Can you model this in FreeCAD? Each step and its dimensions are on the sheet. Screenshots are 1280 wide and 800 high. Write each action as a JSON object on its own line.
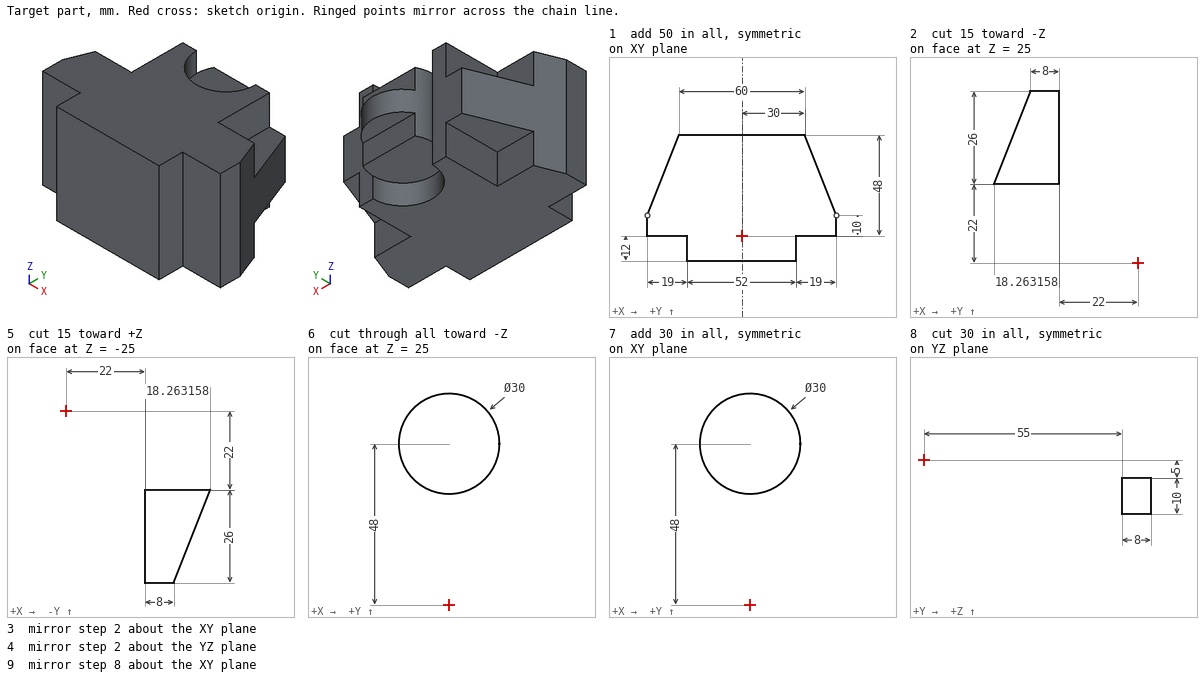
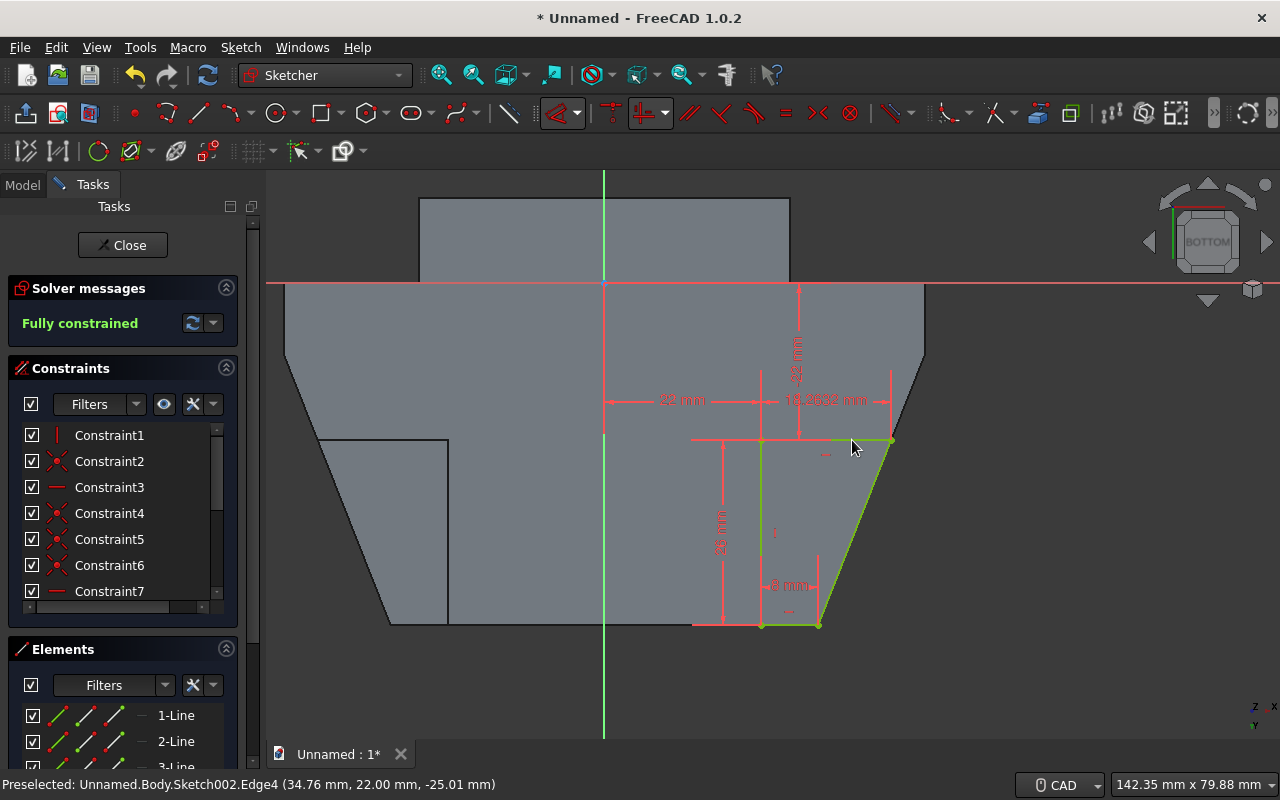
{"action": "left_click", "coordinate": [123, 245]}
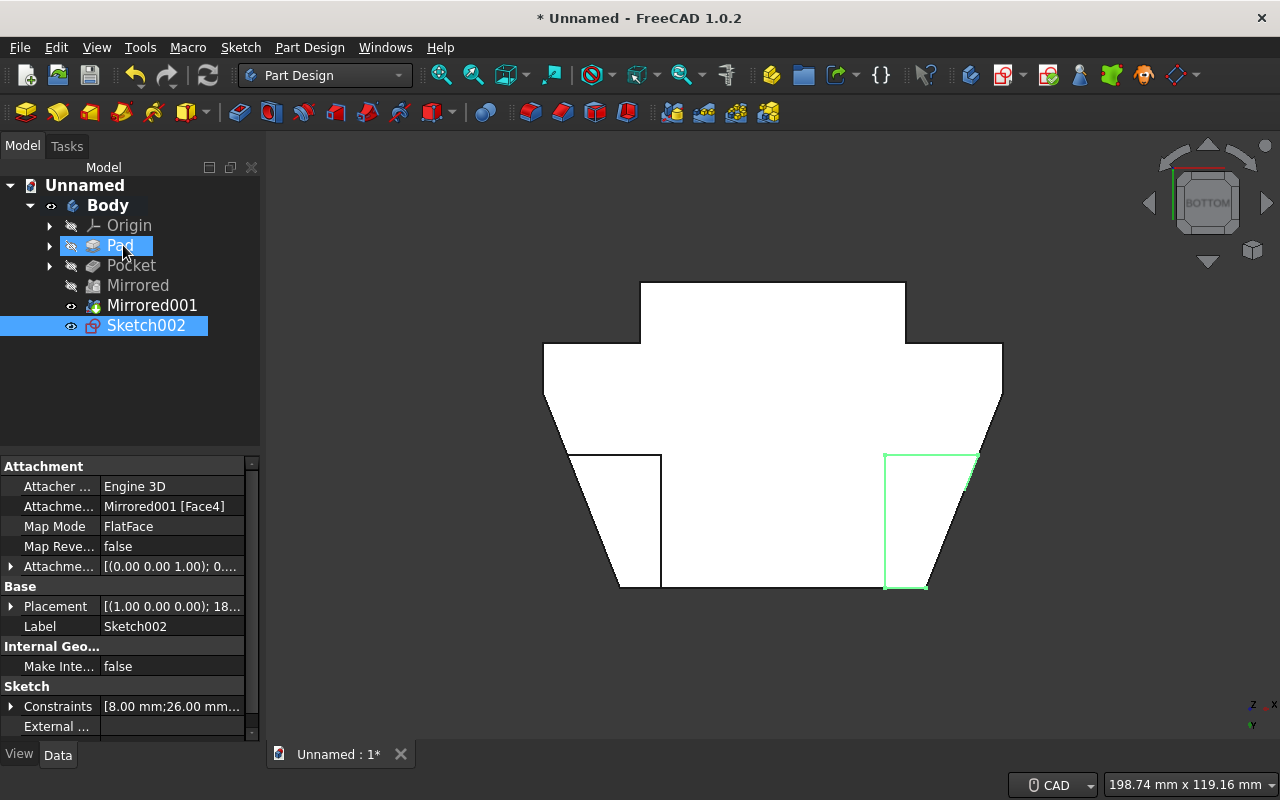
{"action": "left_click", "coordinate": [240, 112]}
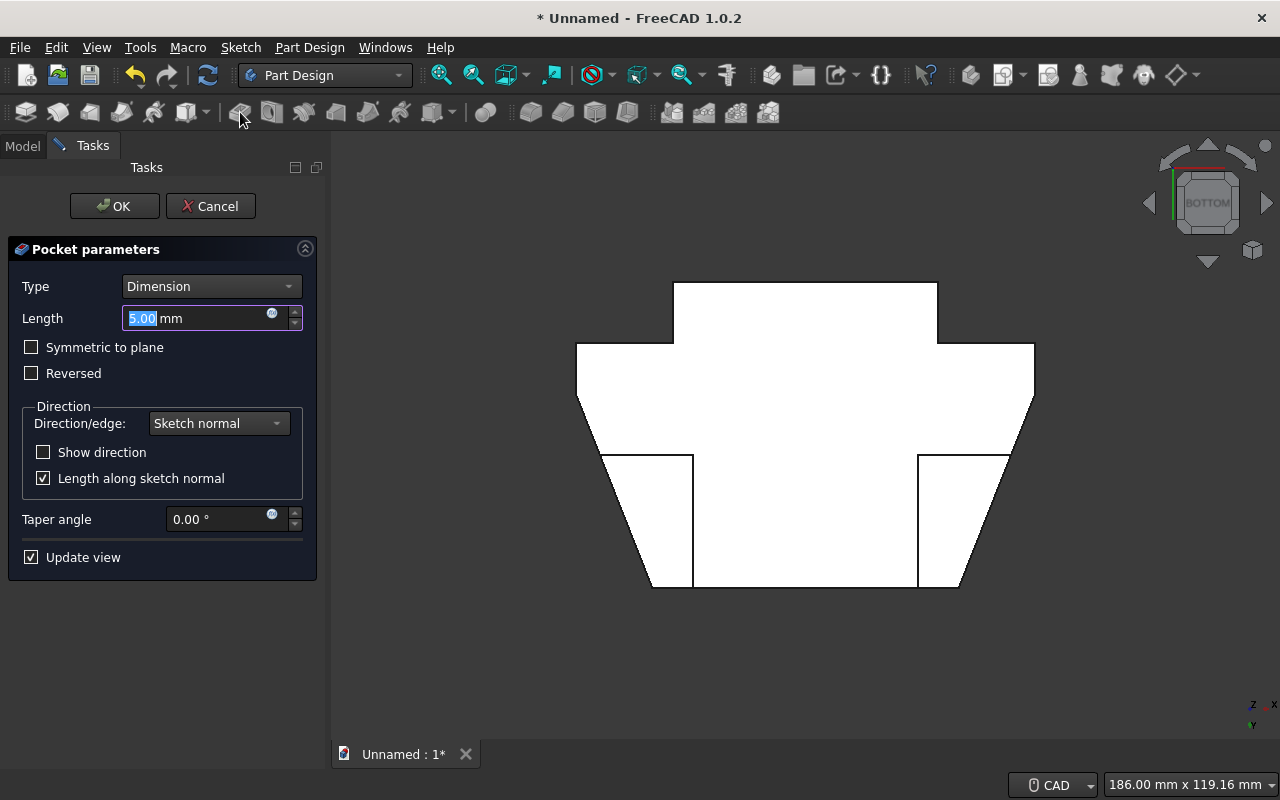
{"action": "type", "text": "15"}
{"action": "key", "text": "Tab"}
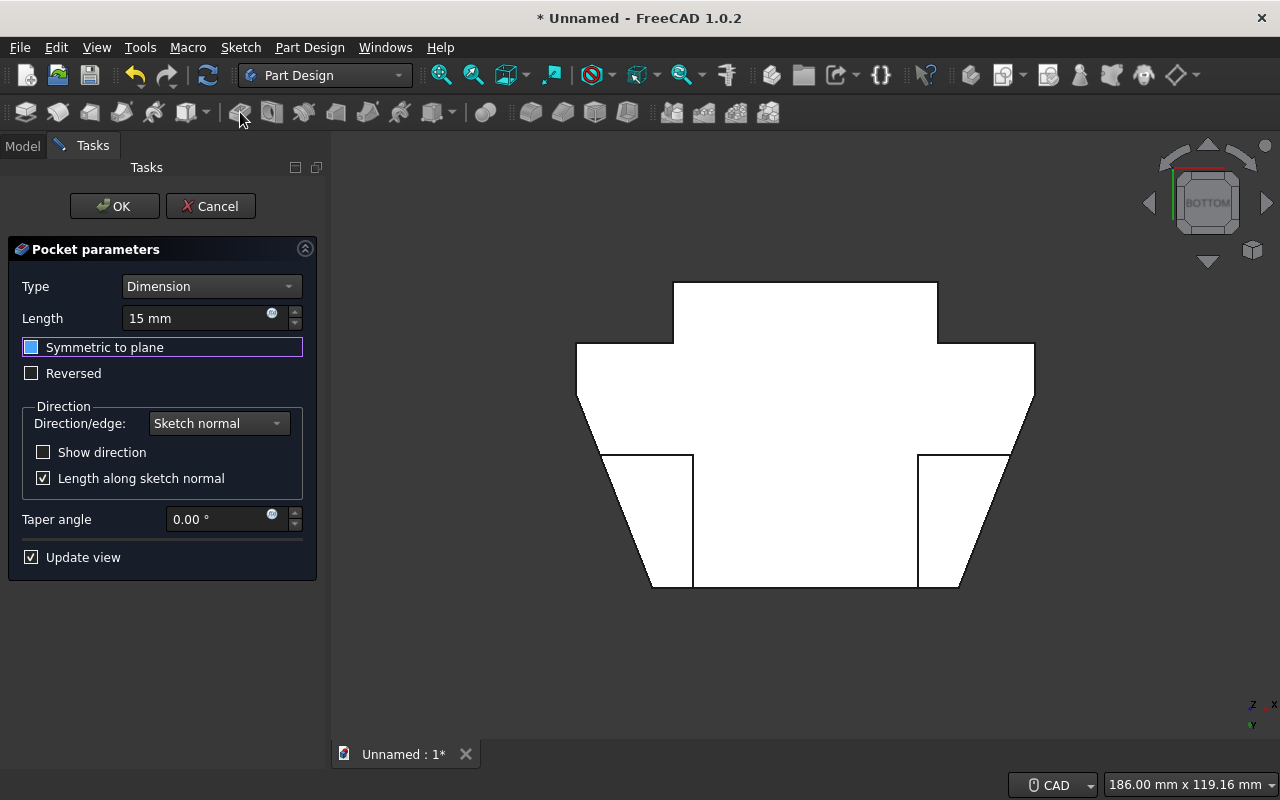
{"action": "left_click", "coordinate": [115, 206]}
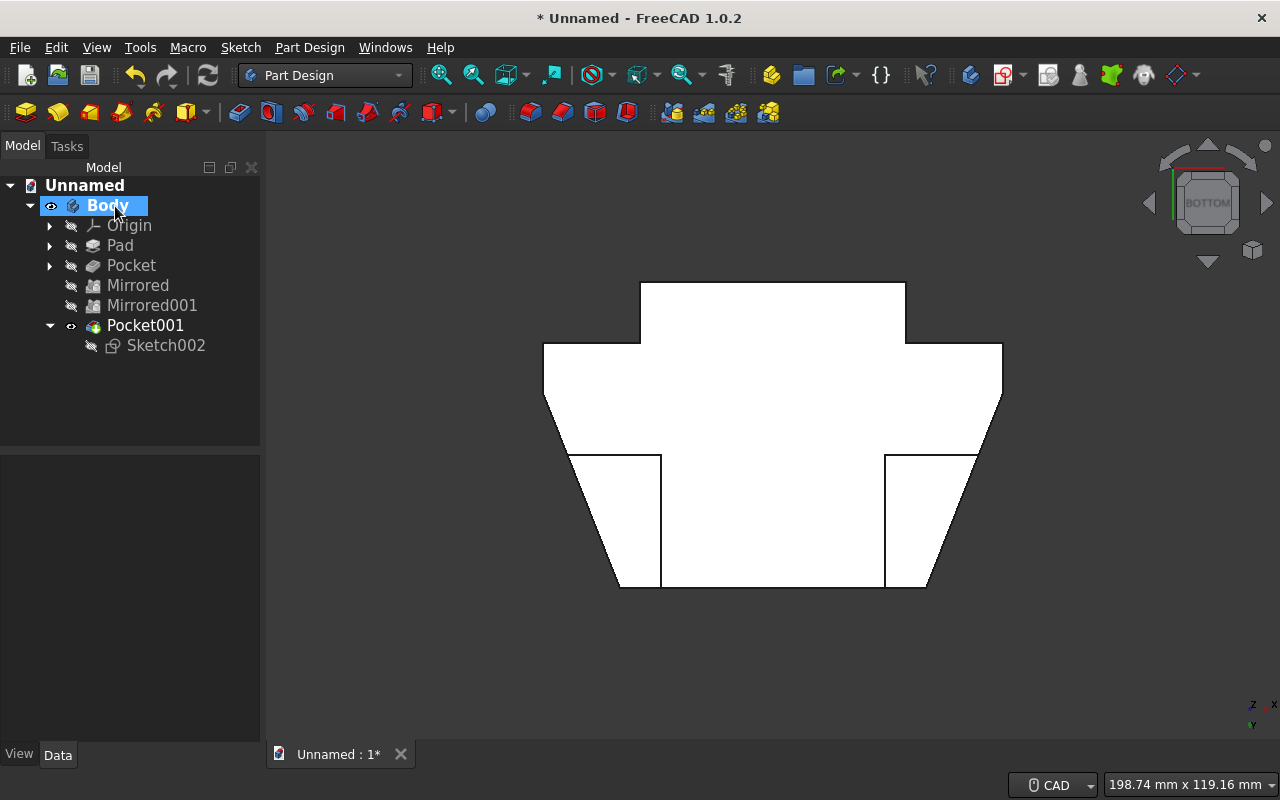
{"action": "key", "text": "0"}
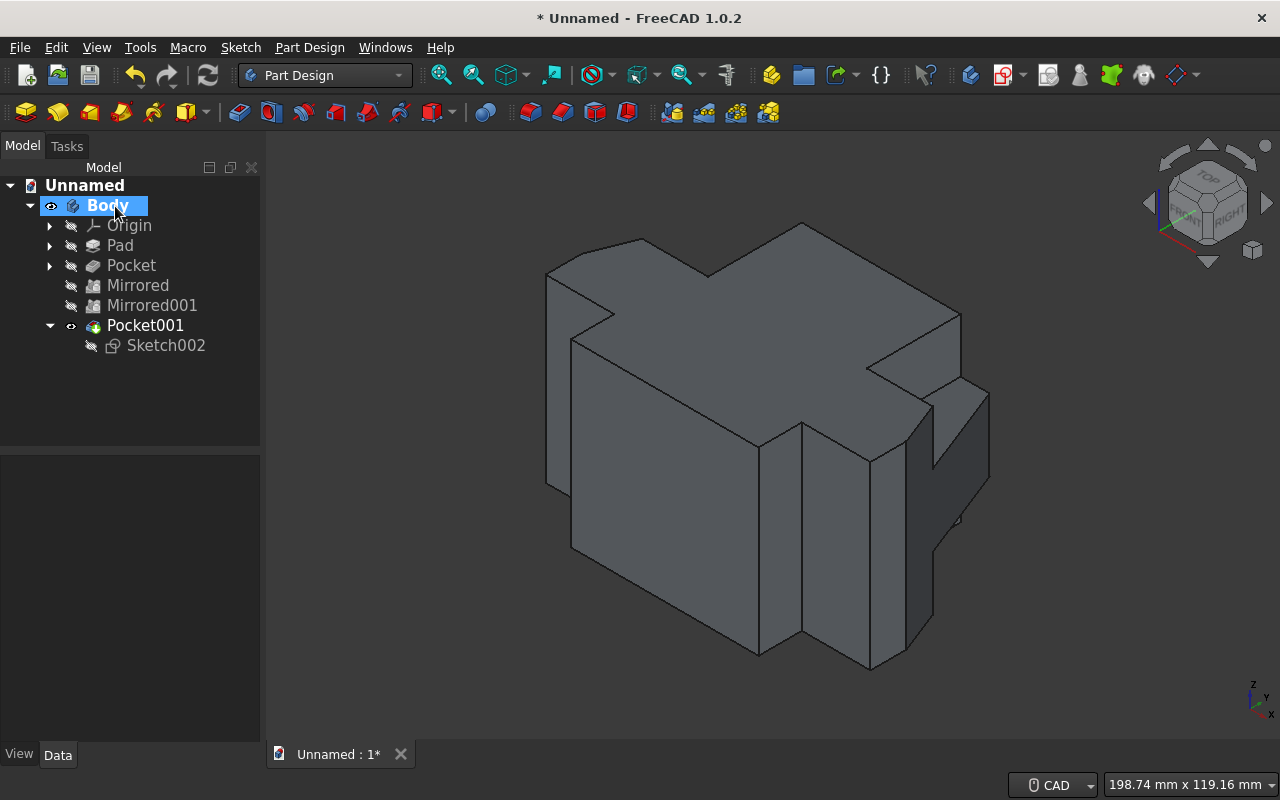
{"action": "left_click", "coordinate": [773, 330]}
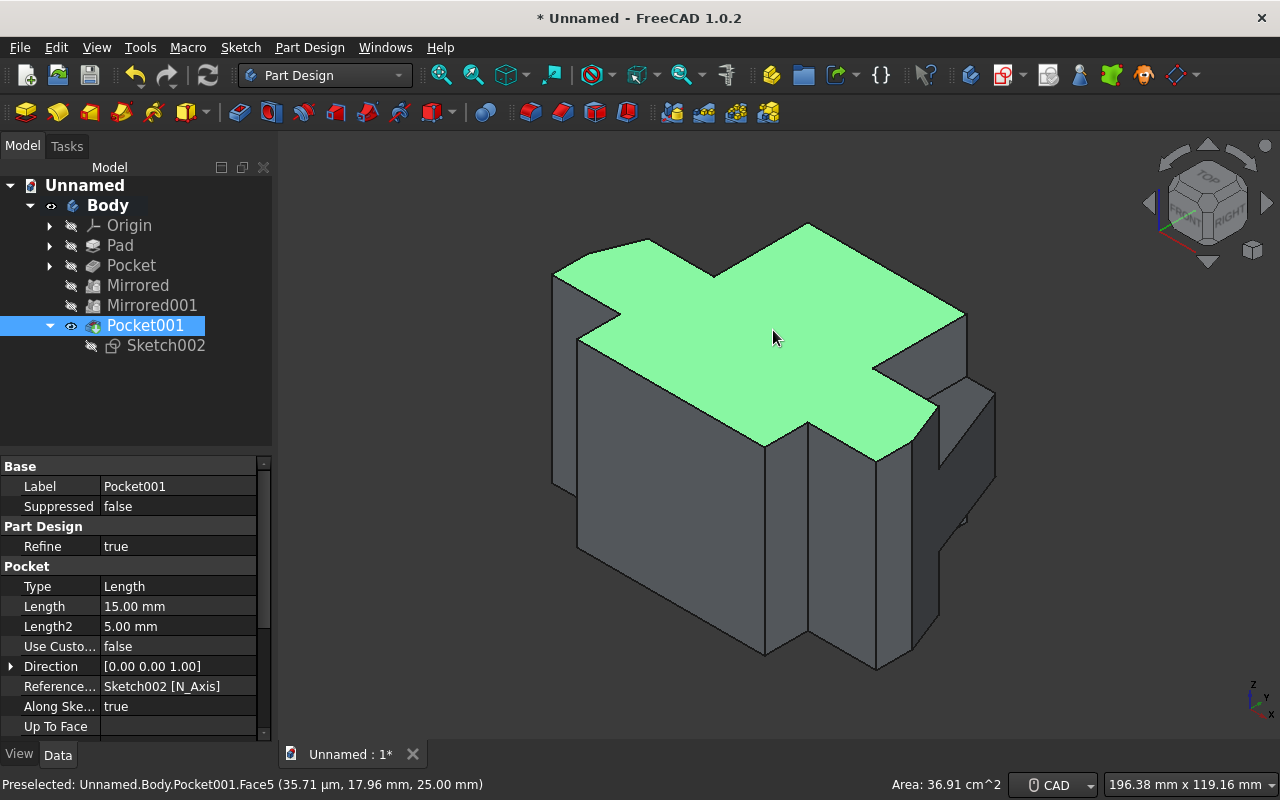
{"action": "left_click", "coordinate": [1004, 76]}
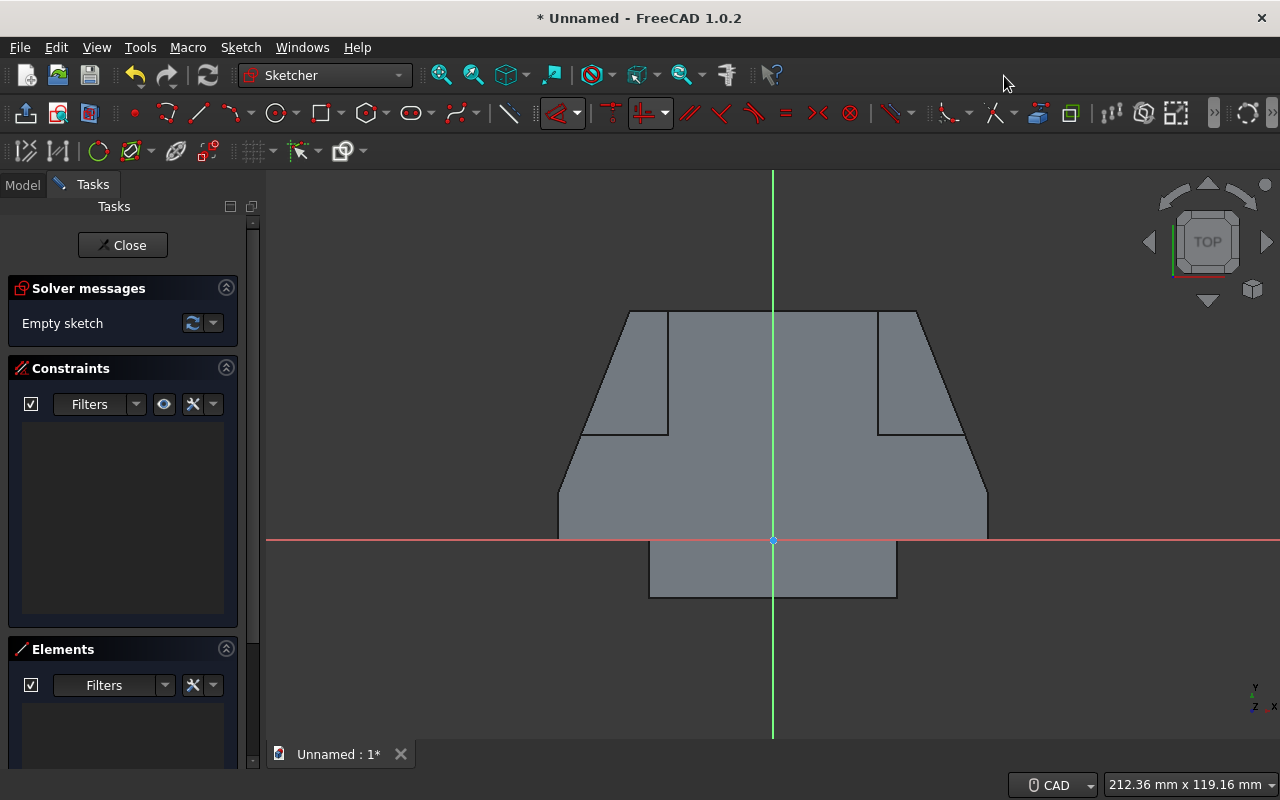
{"action": "left_click", "coordinate": [276, 114]}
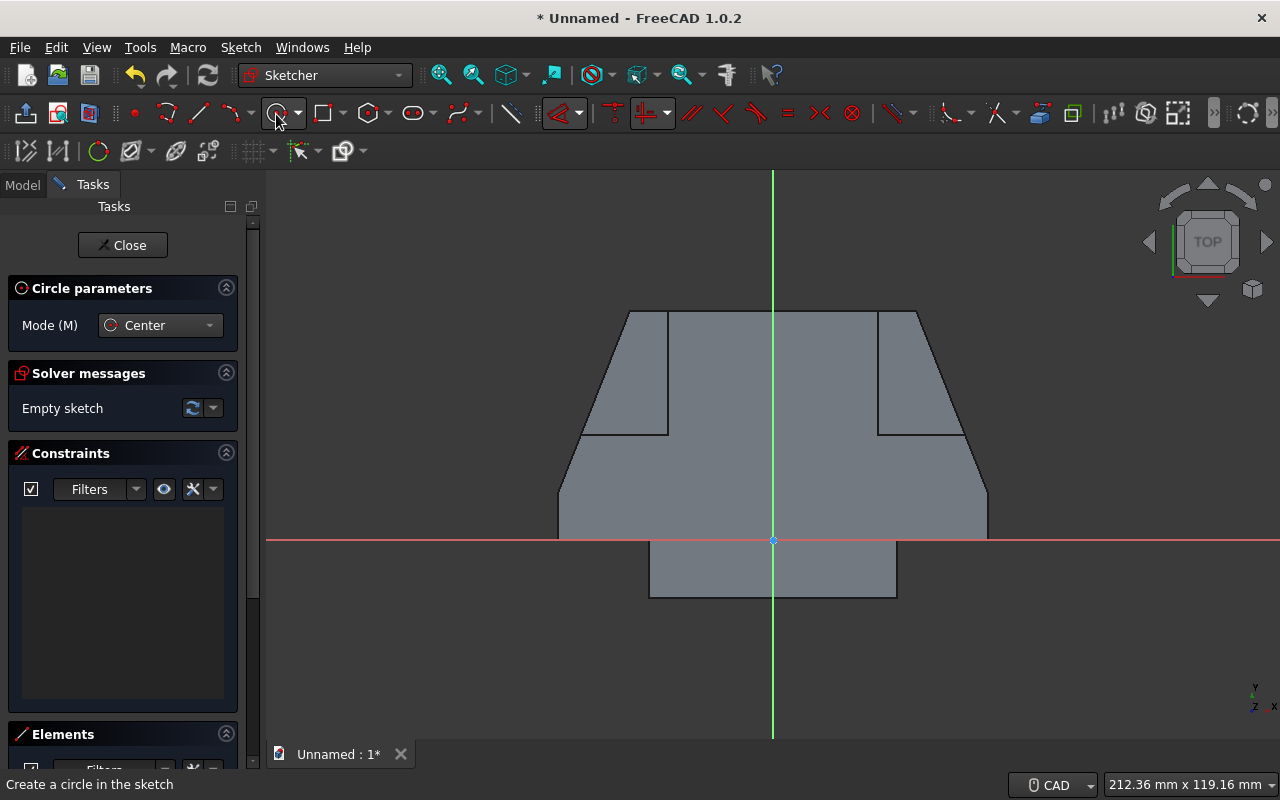
{"action": "left_click", "coordinate": [773, 311]}
{"action": "left_click", "coordinate": [824, 261]}
{"action": "key", "text": "Escape"}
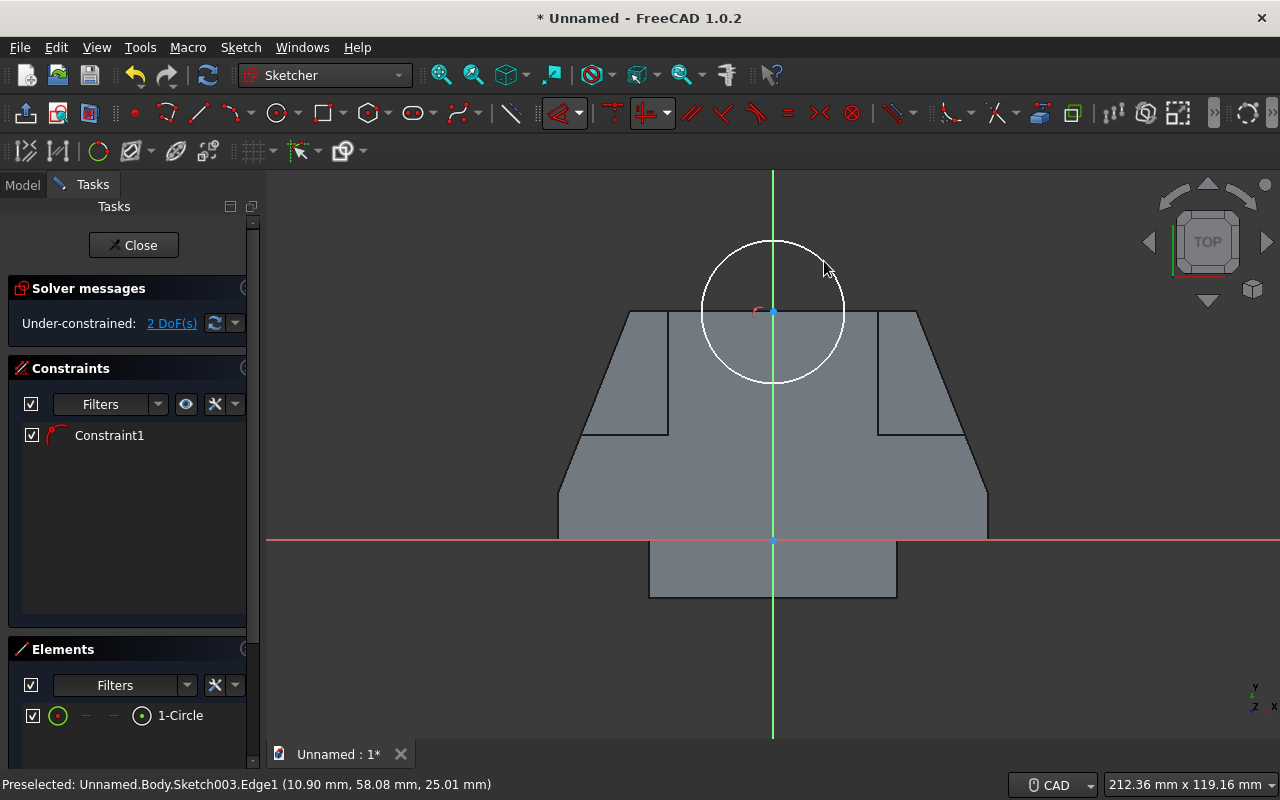
{"action": "left_click", "coordinate": [823, 261]}